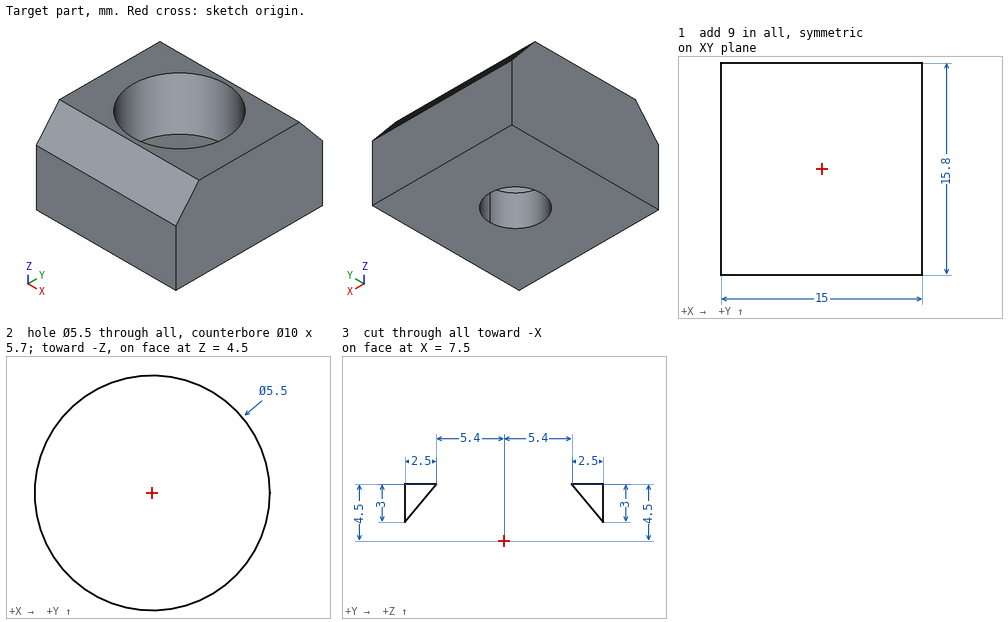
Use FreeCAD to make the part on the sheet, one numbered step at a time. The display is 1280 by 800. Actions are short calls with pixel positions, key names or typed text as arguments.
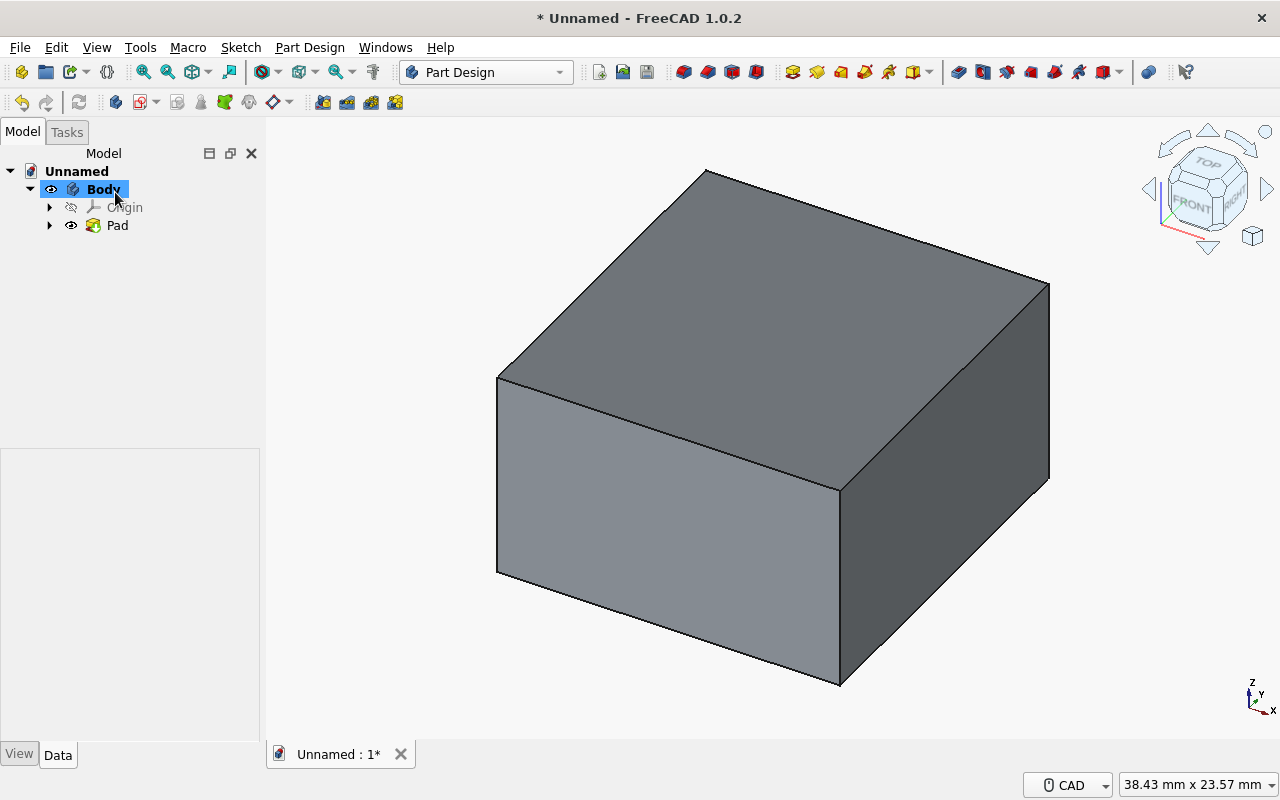
click(773, 330)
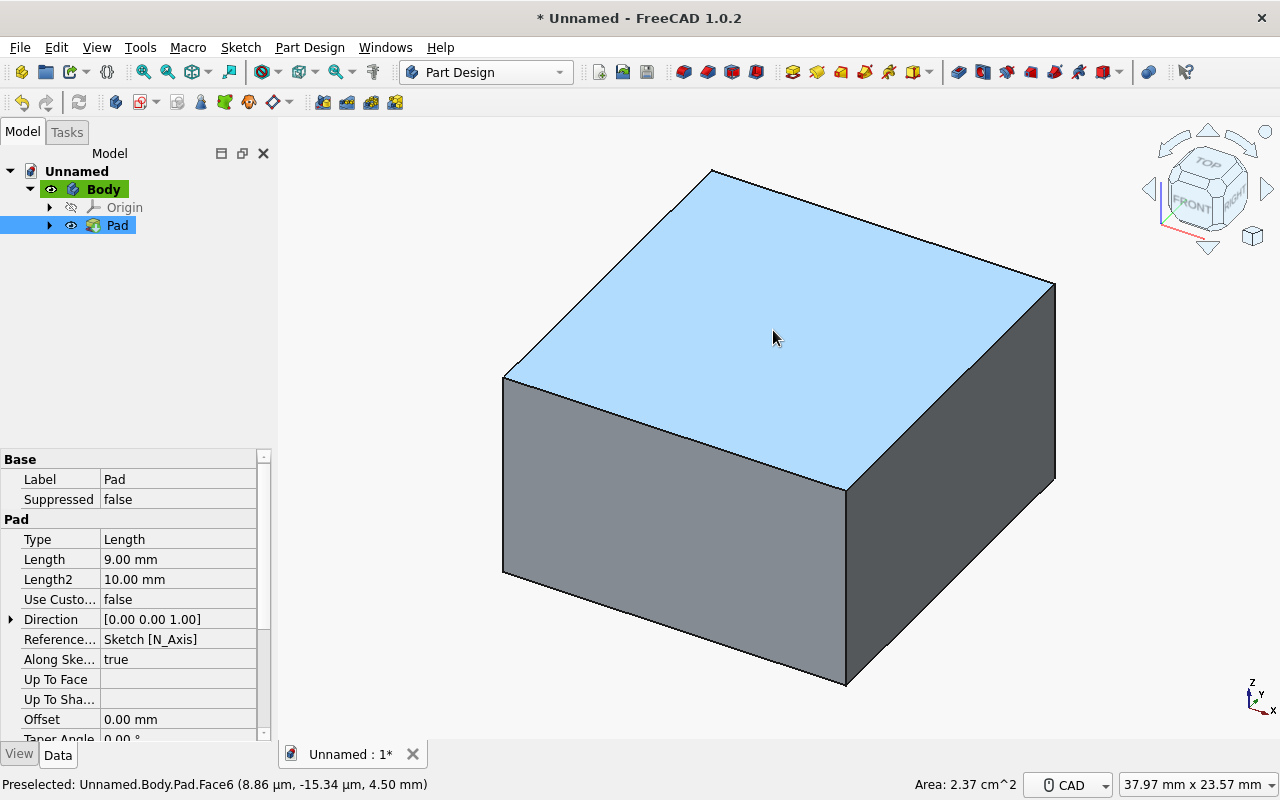
click(140, 102)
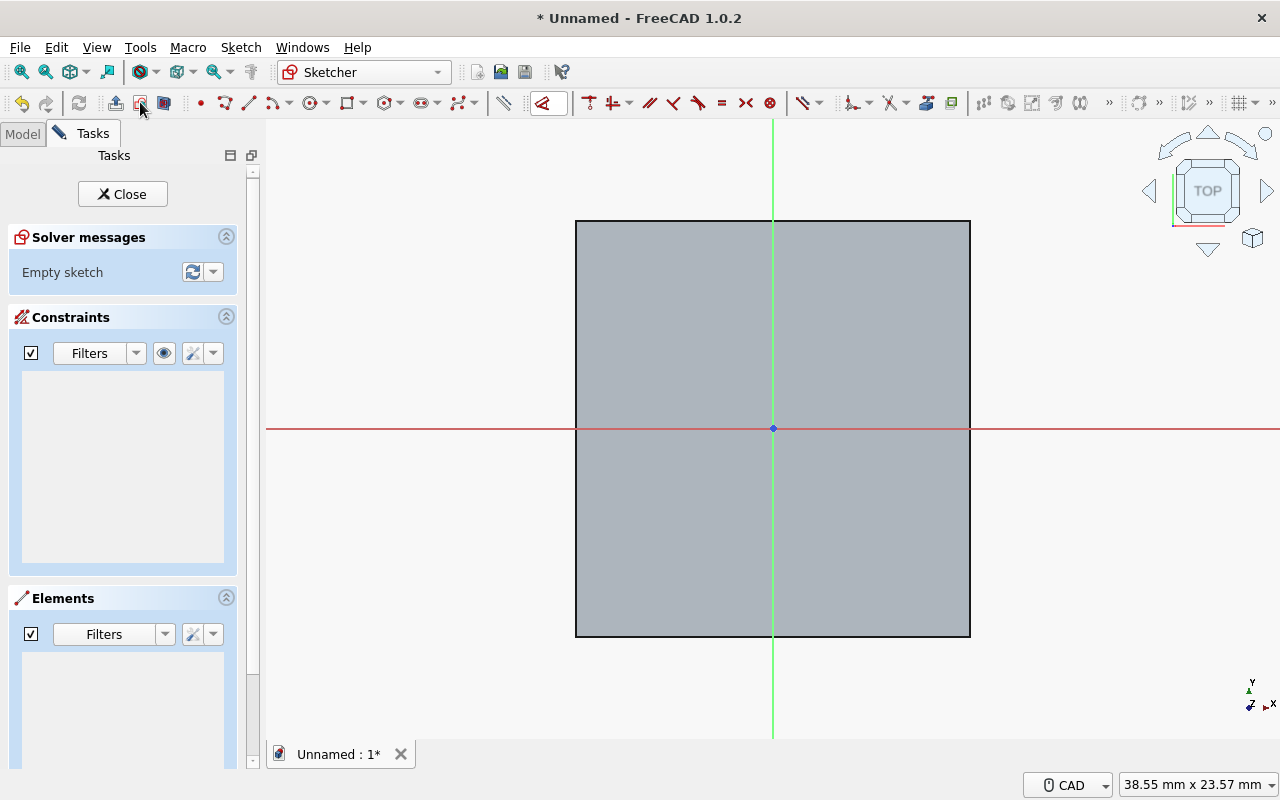
scroll(813, 429, up, 5)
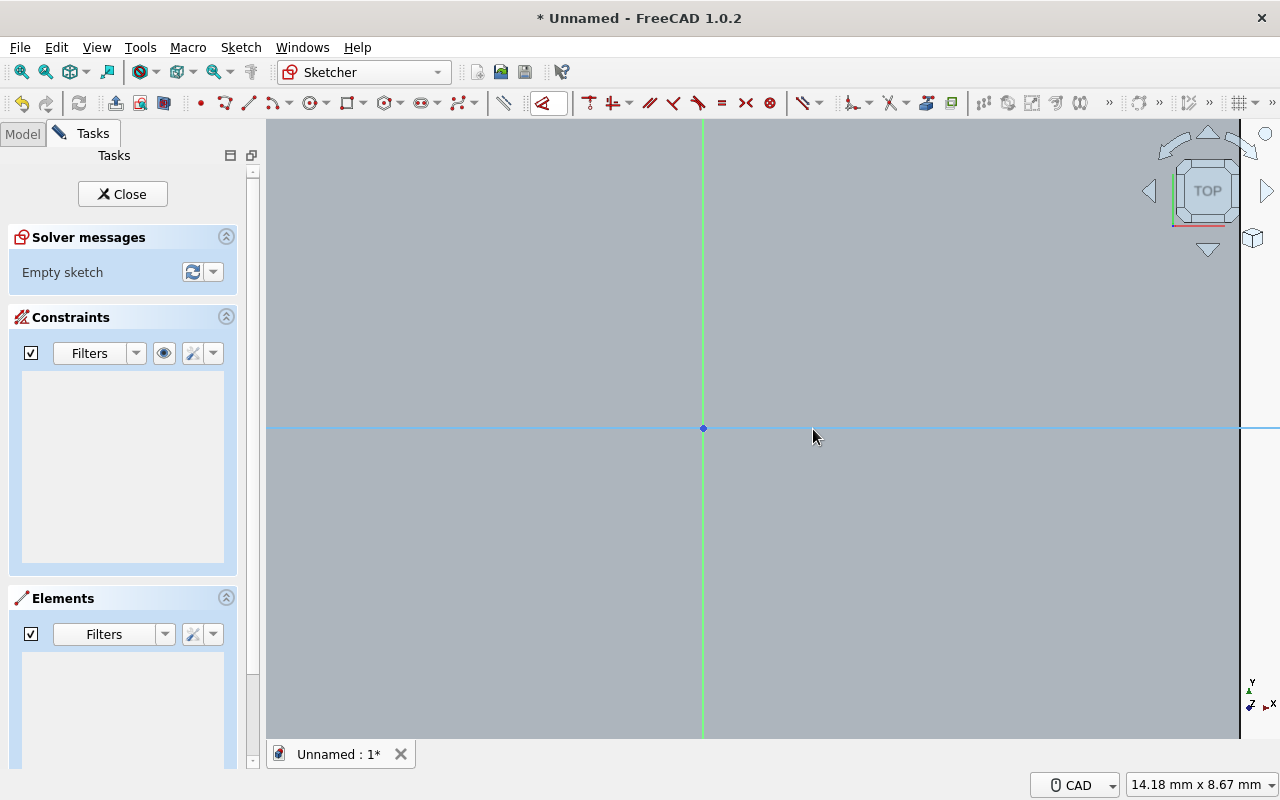
click(310, 104)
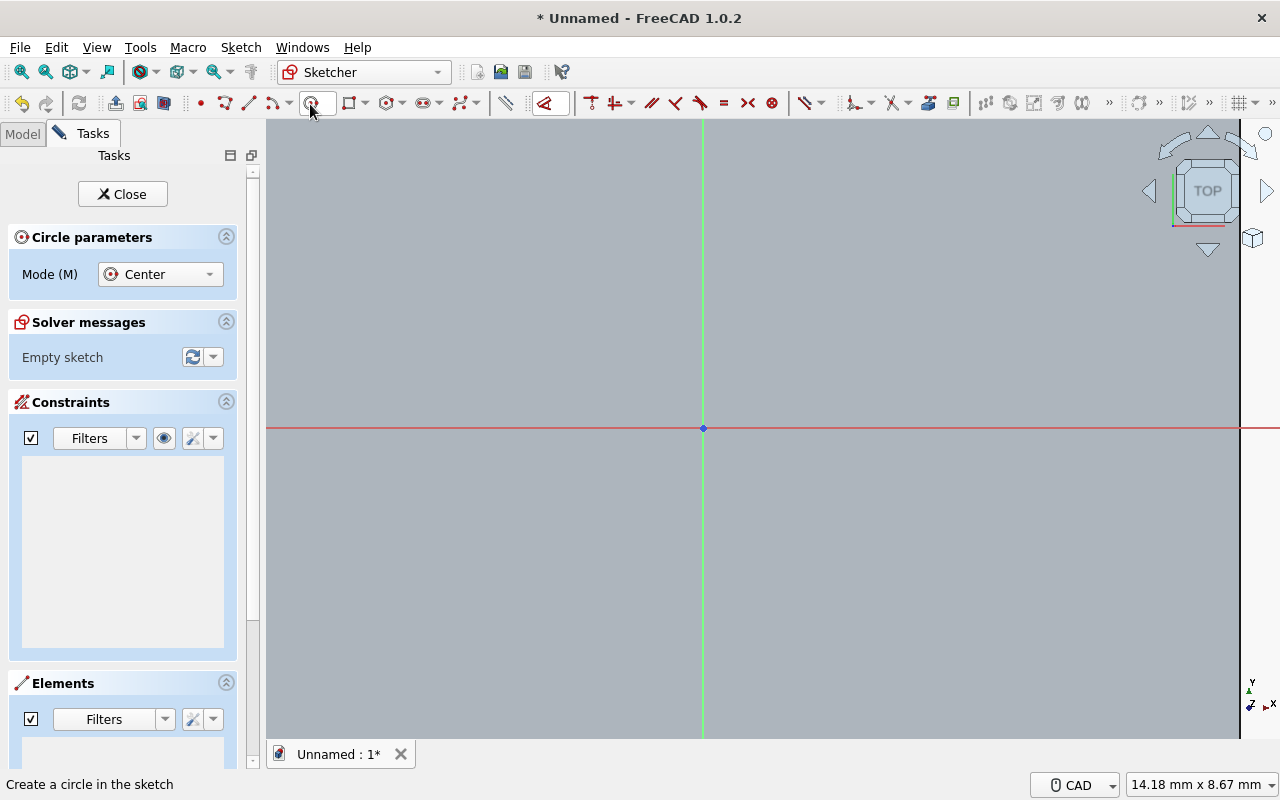
click(703, 428)
click(842, 289)
key(Escape)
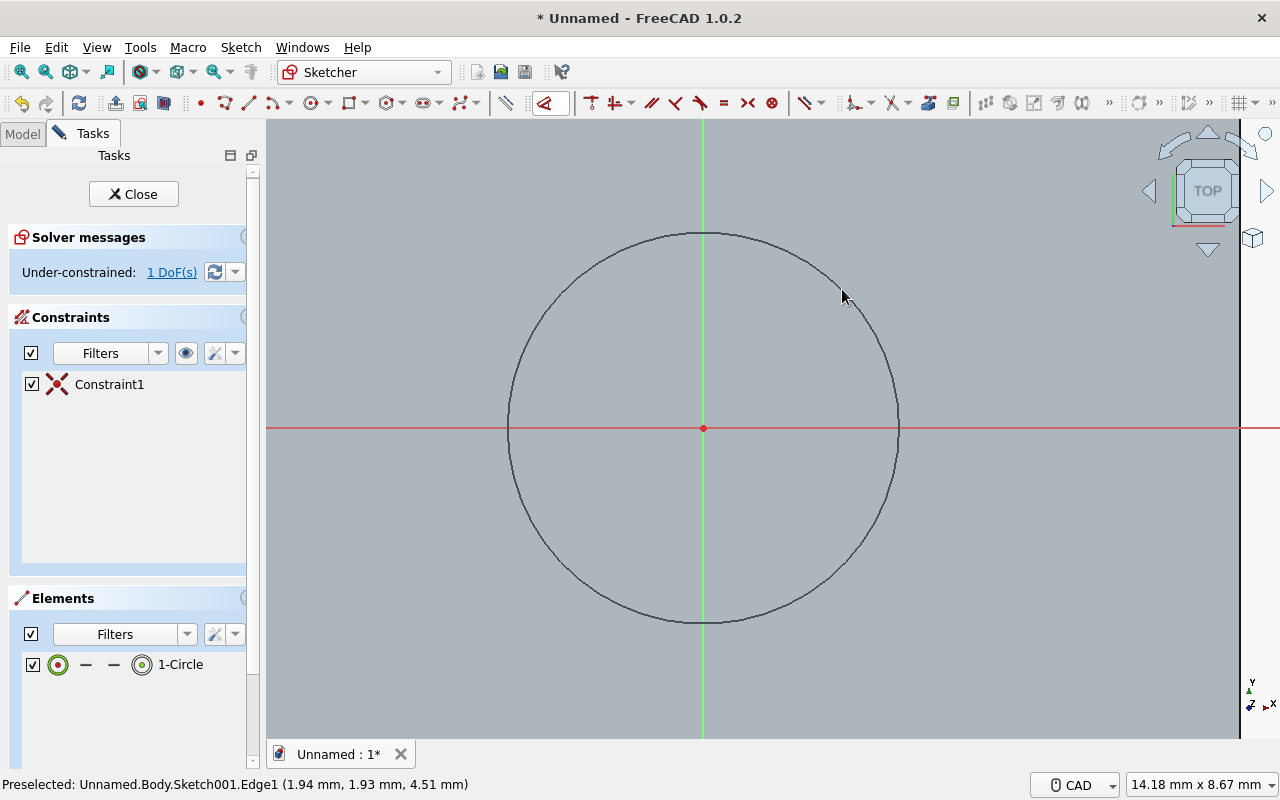
click(841, 289)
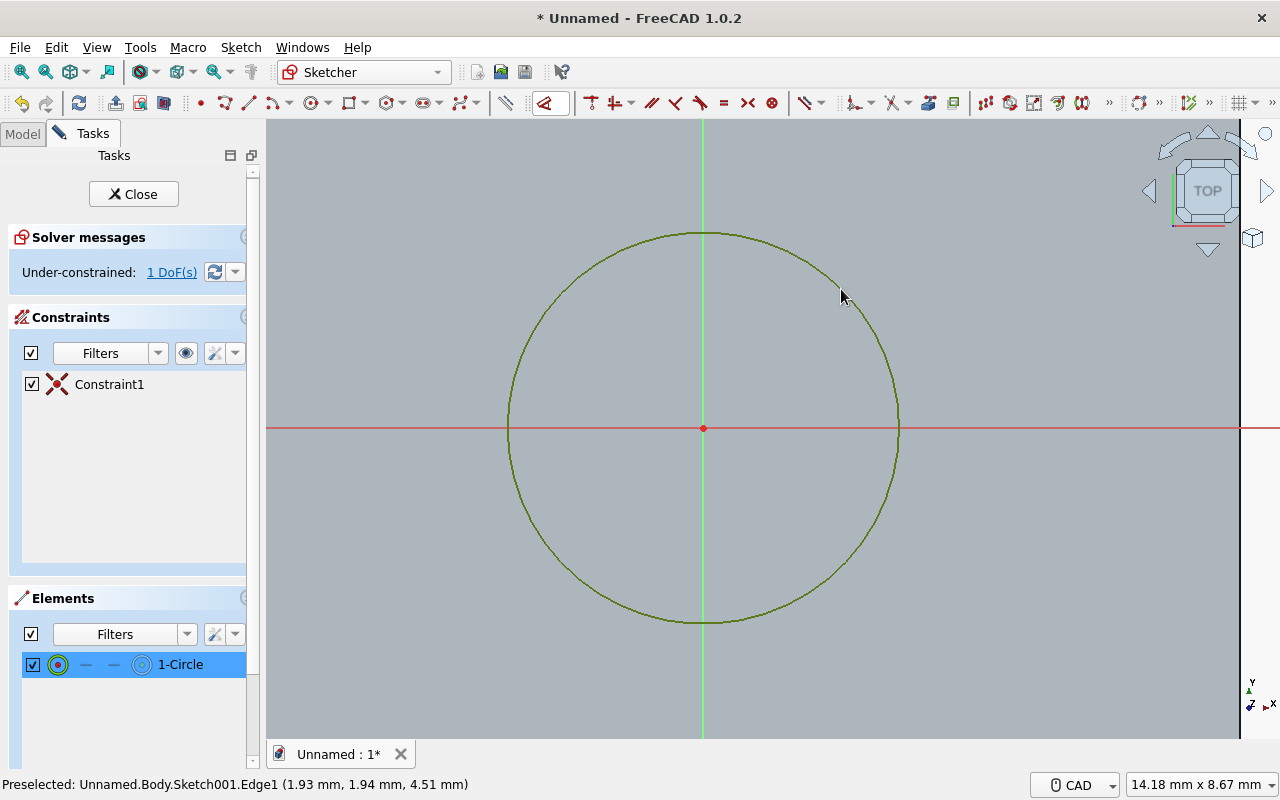
key(k)
key(o)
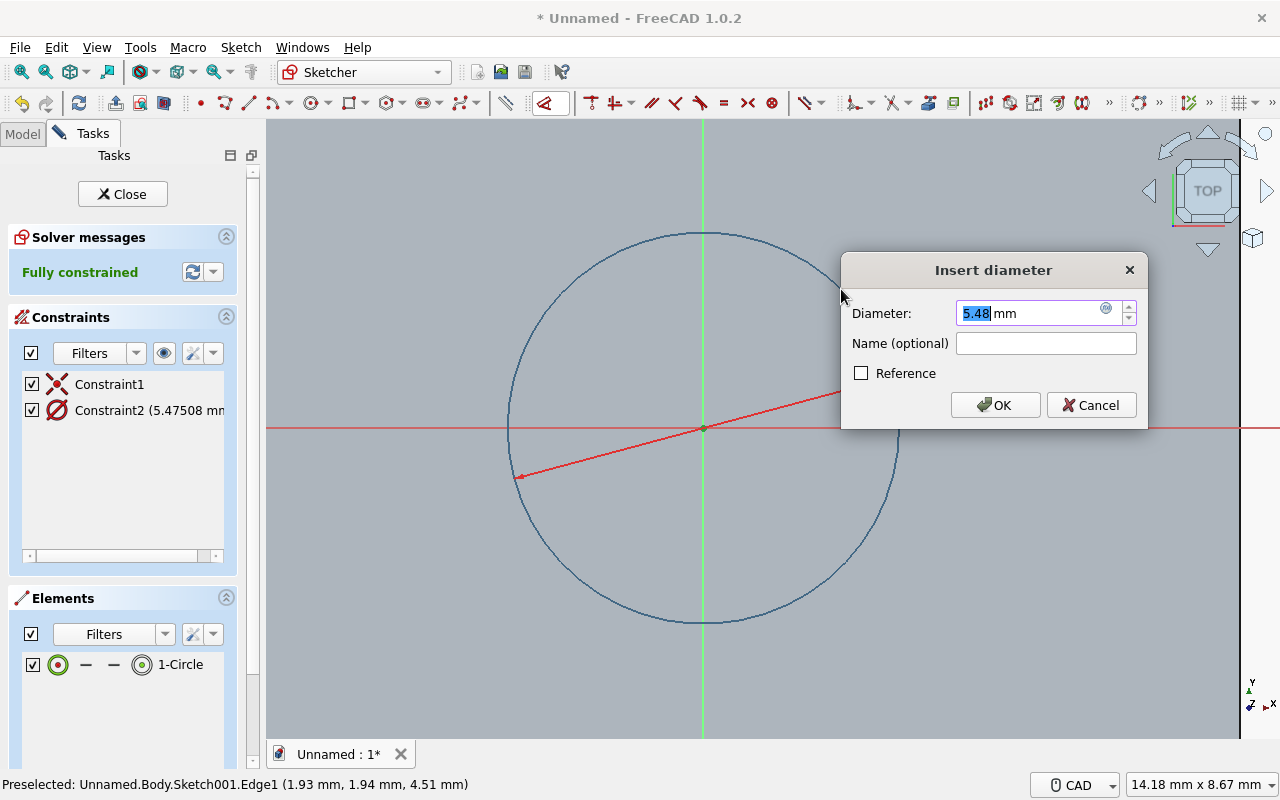
text(5.5)
key(Return)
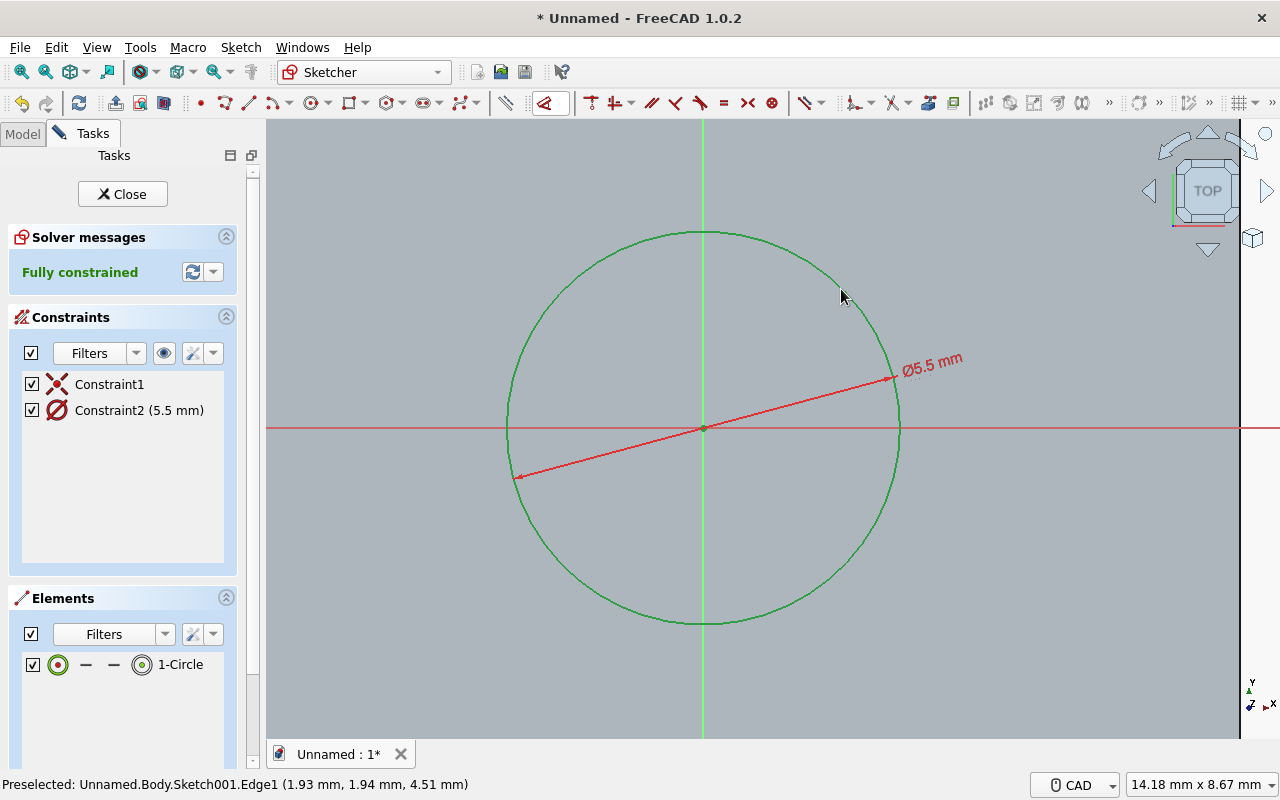
click(123, 194)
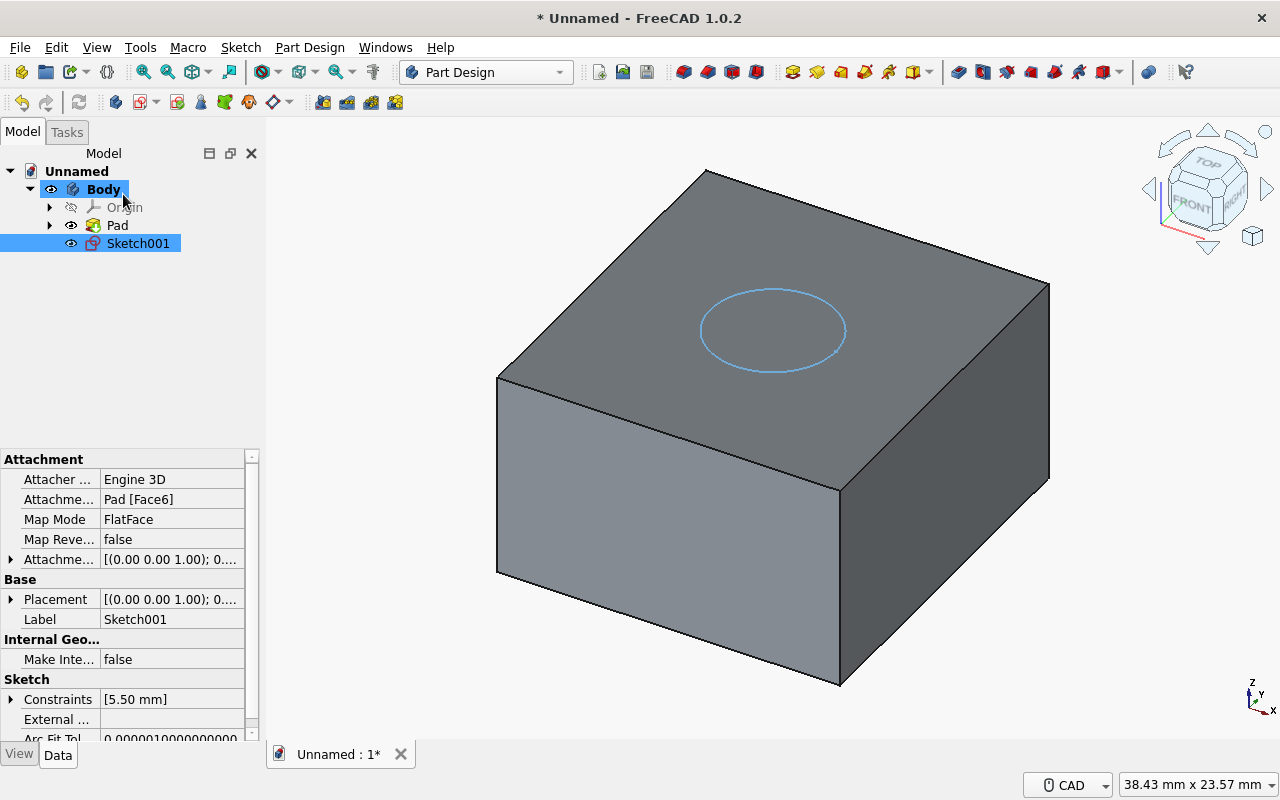
click(984, 72)